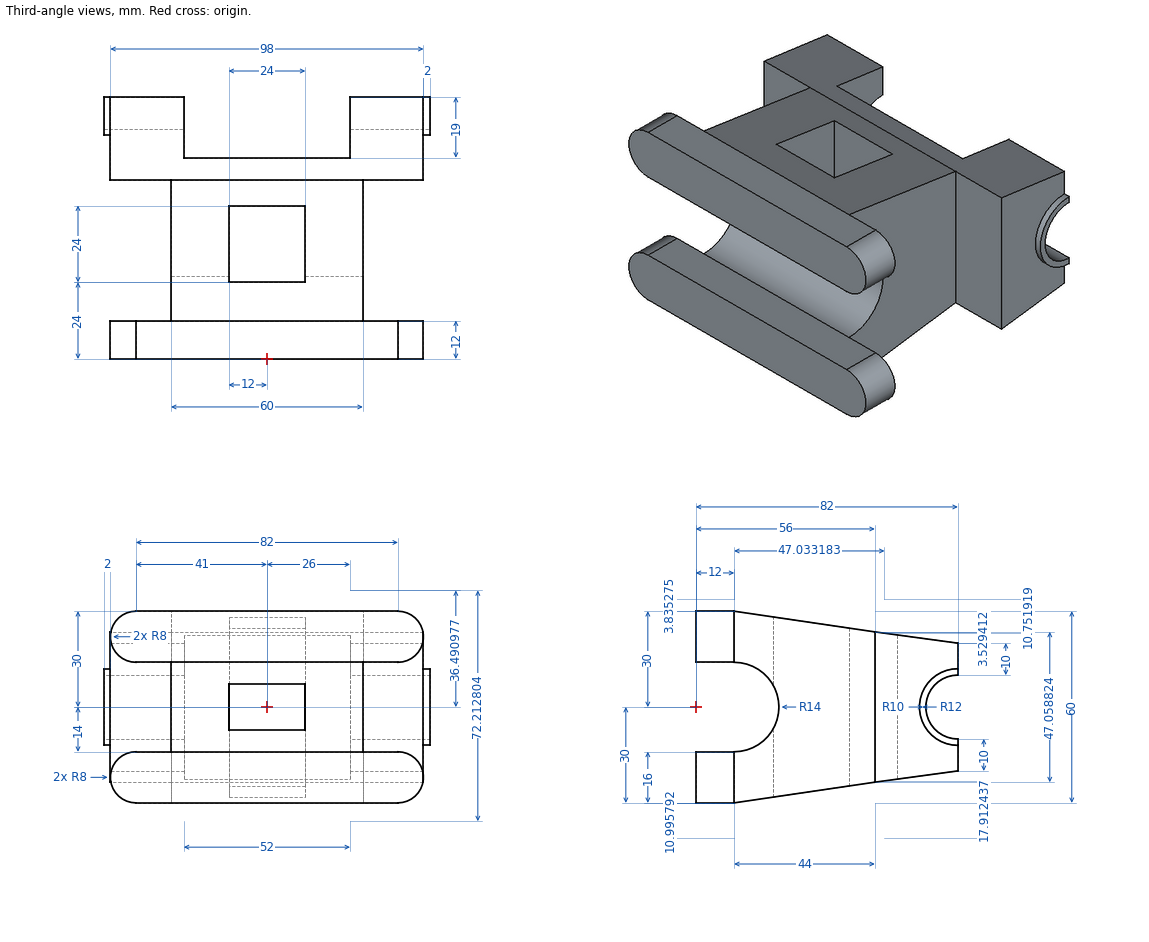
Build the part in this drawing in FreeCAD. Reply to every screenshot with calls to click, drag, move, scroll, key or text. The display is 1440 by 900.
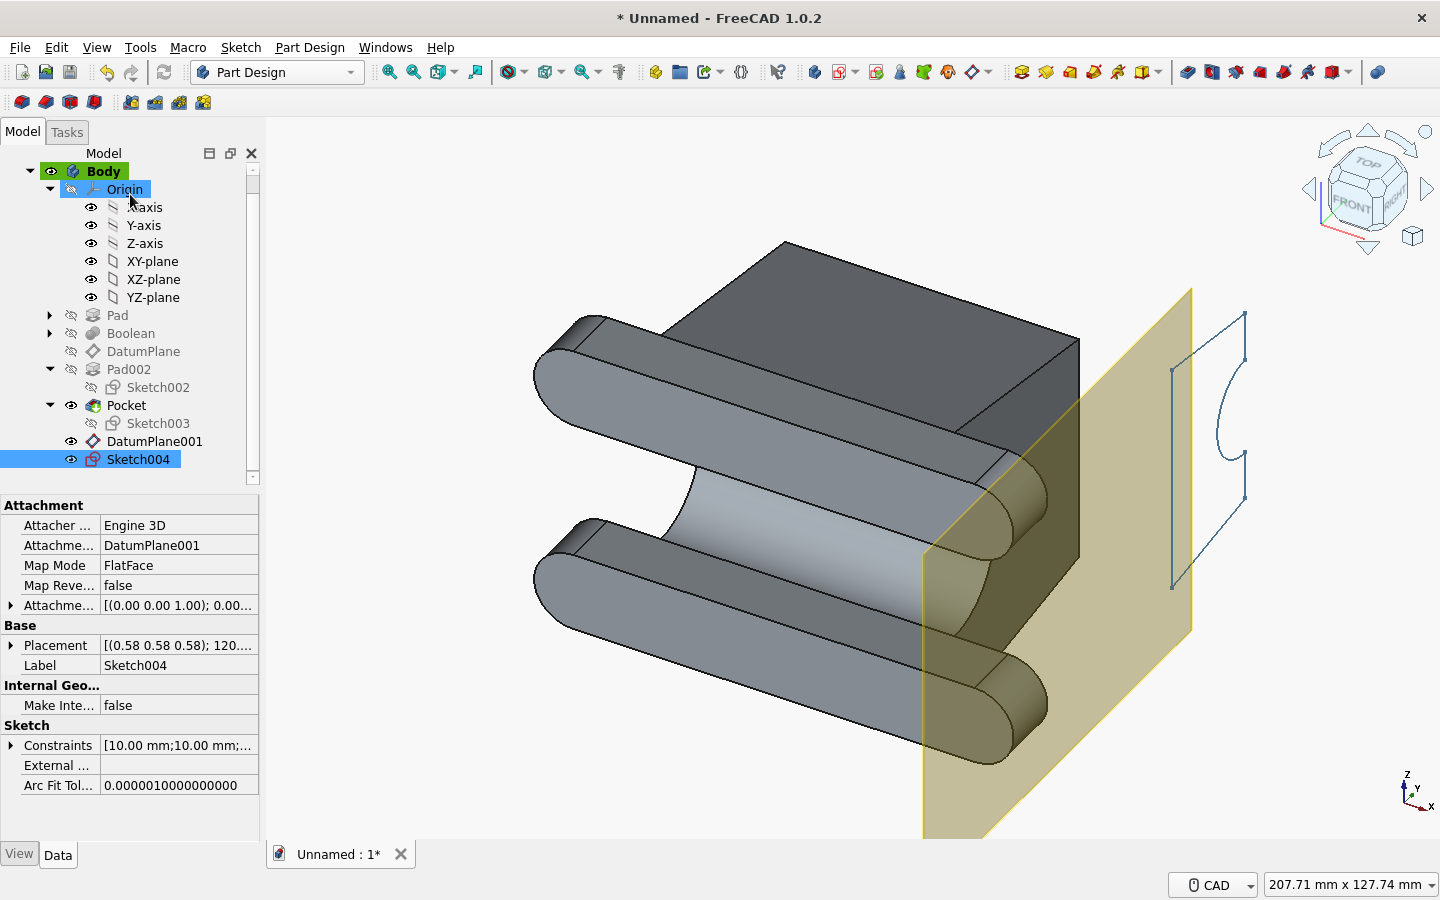
click(1022, 72)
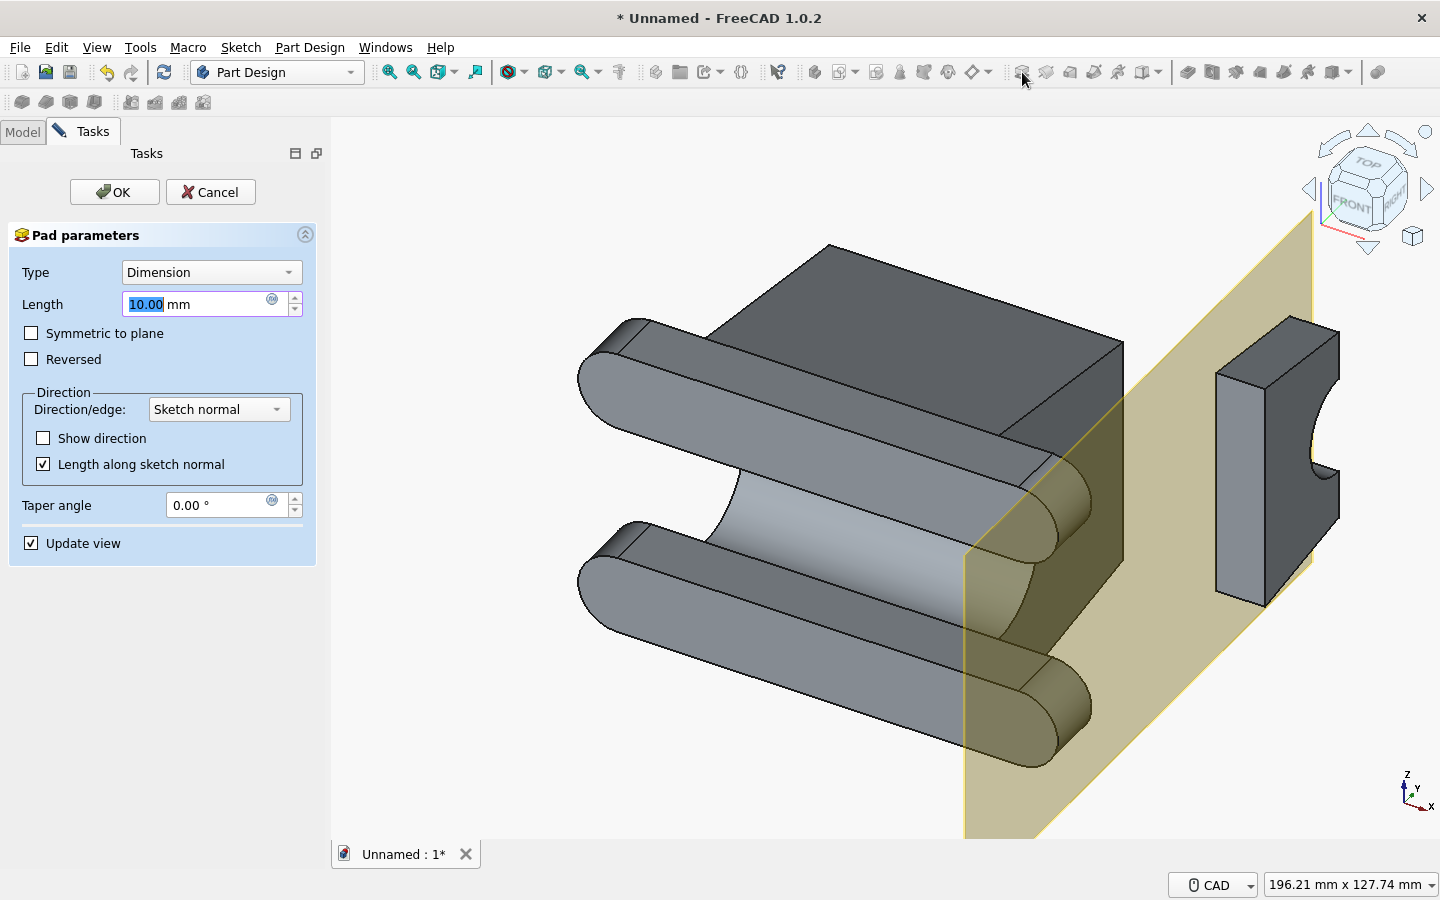
text(98)
key(Tab)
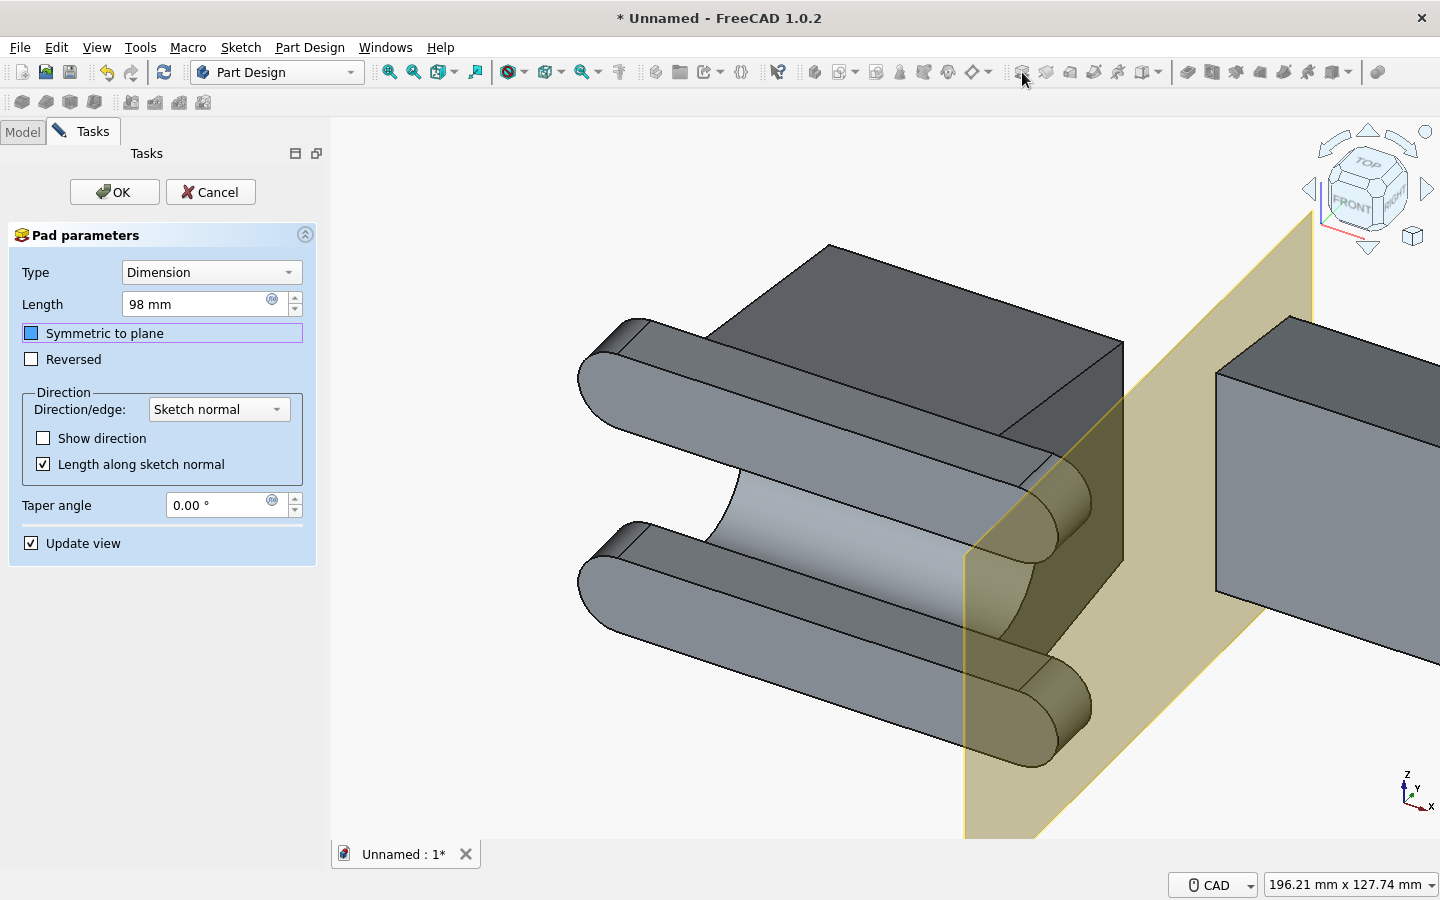
click(30, 359)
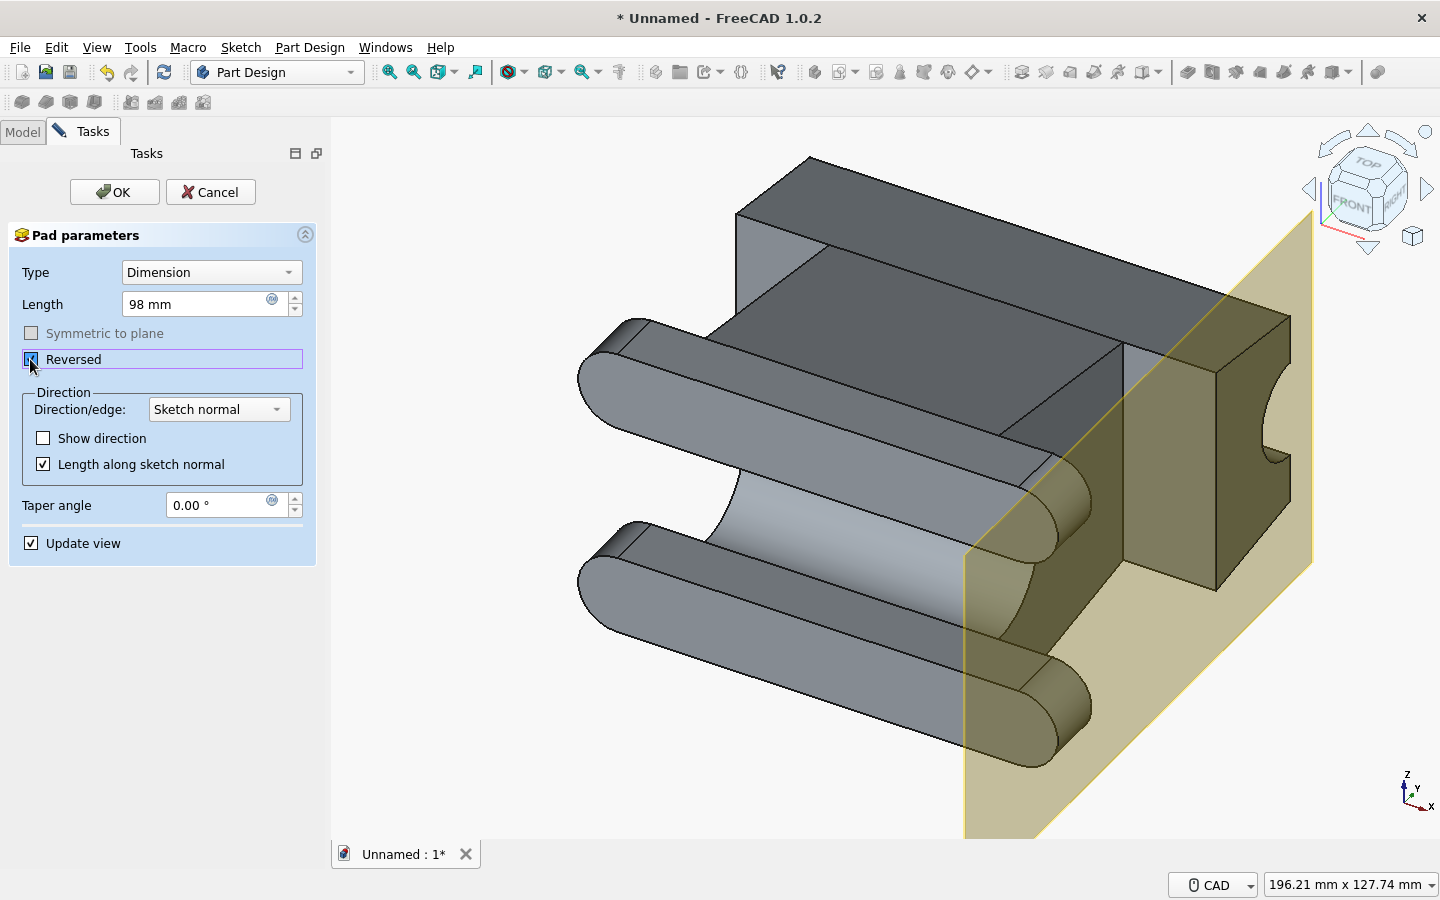
click(115, 192)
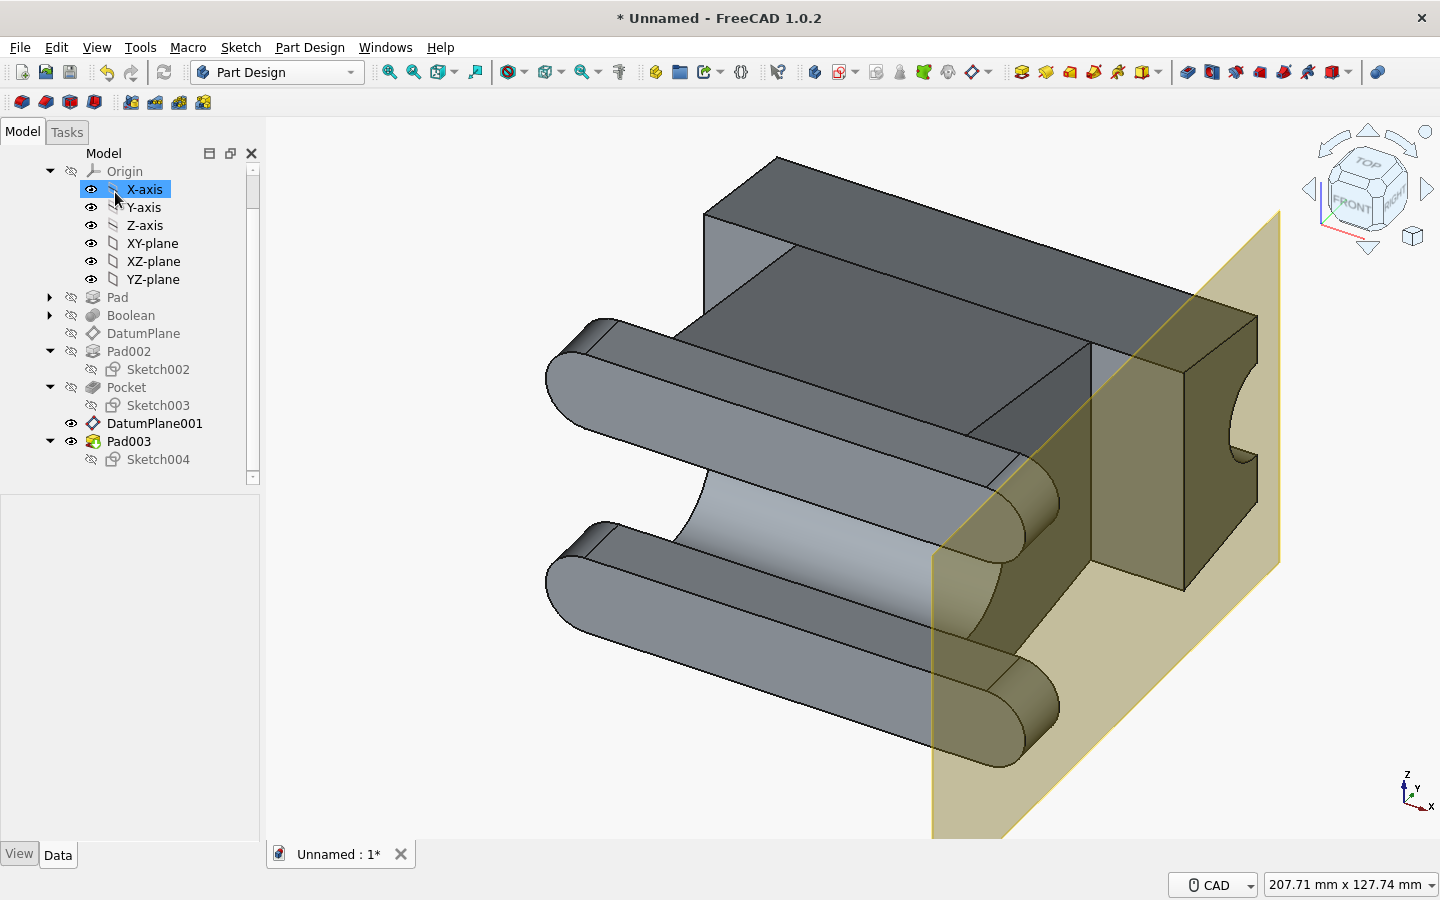
click(116, 423)
key(space)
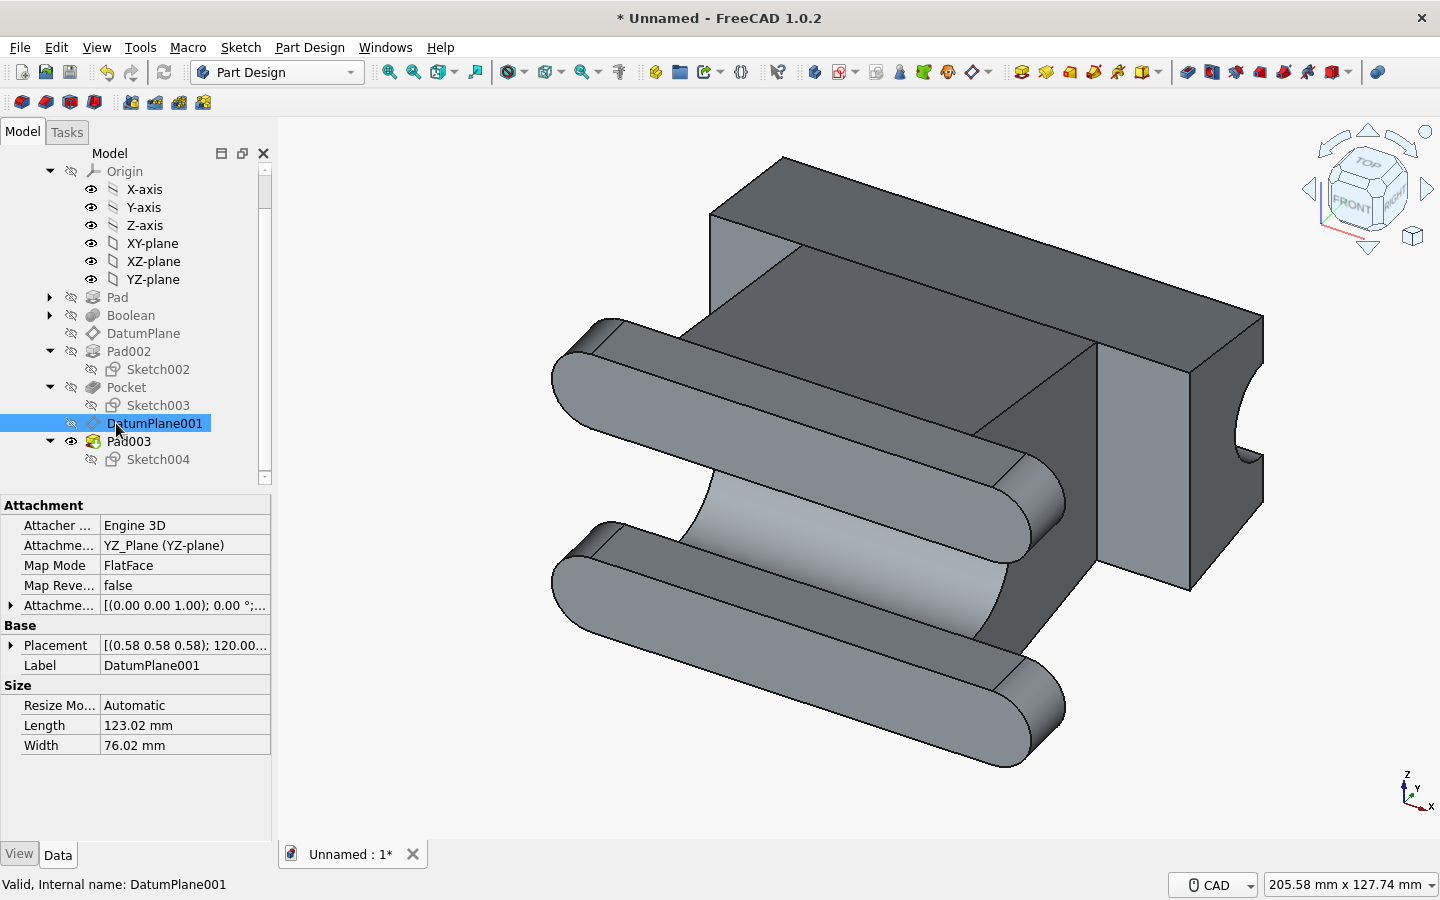
click(390, 72)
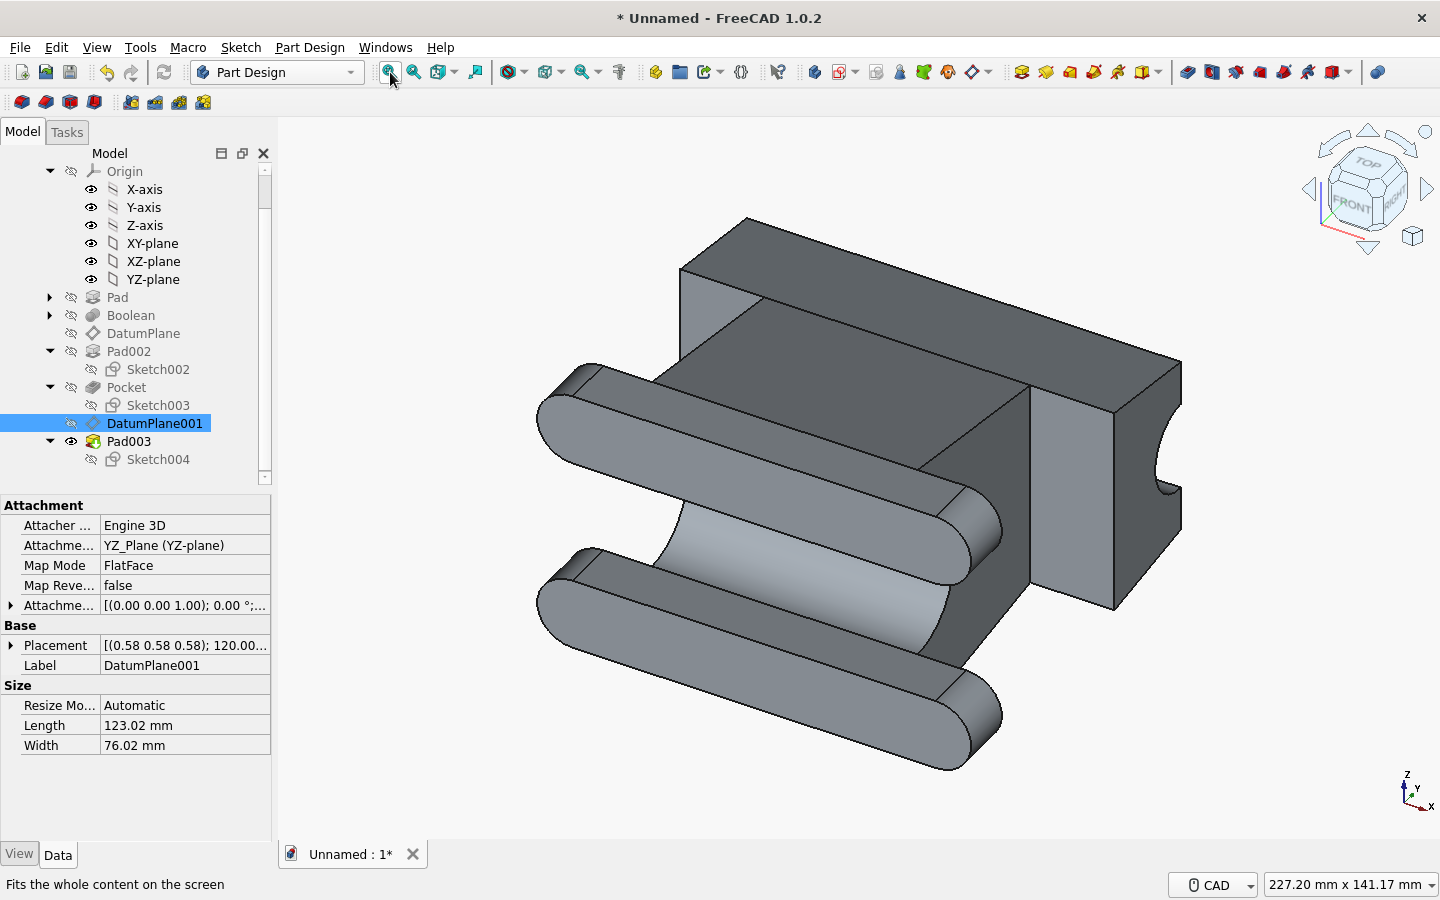
key(4)